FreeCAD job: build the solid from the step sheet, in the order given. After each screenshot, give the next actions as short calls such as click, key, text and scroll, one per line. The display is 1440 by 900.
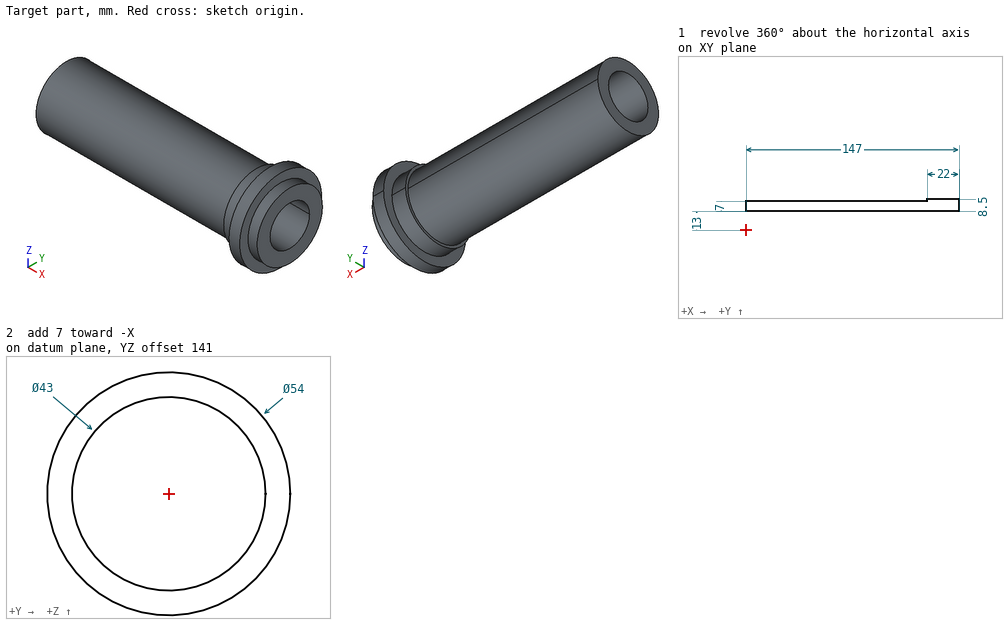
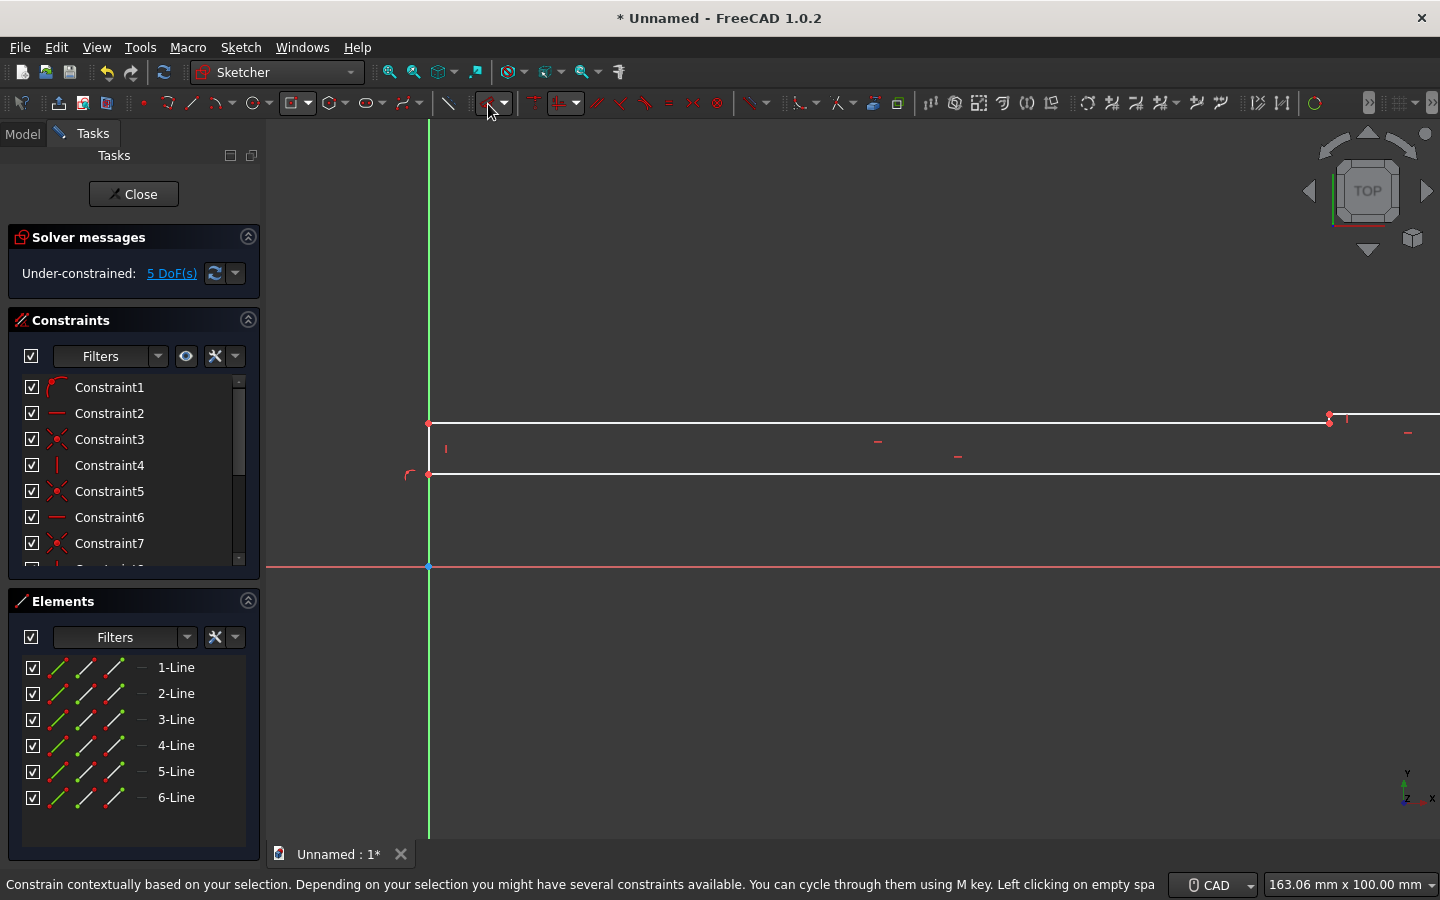
click(429, 438)
click(395, 449)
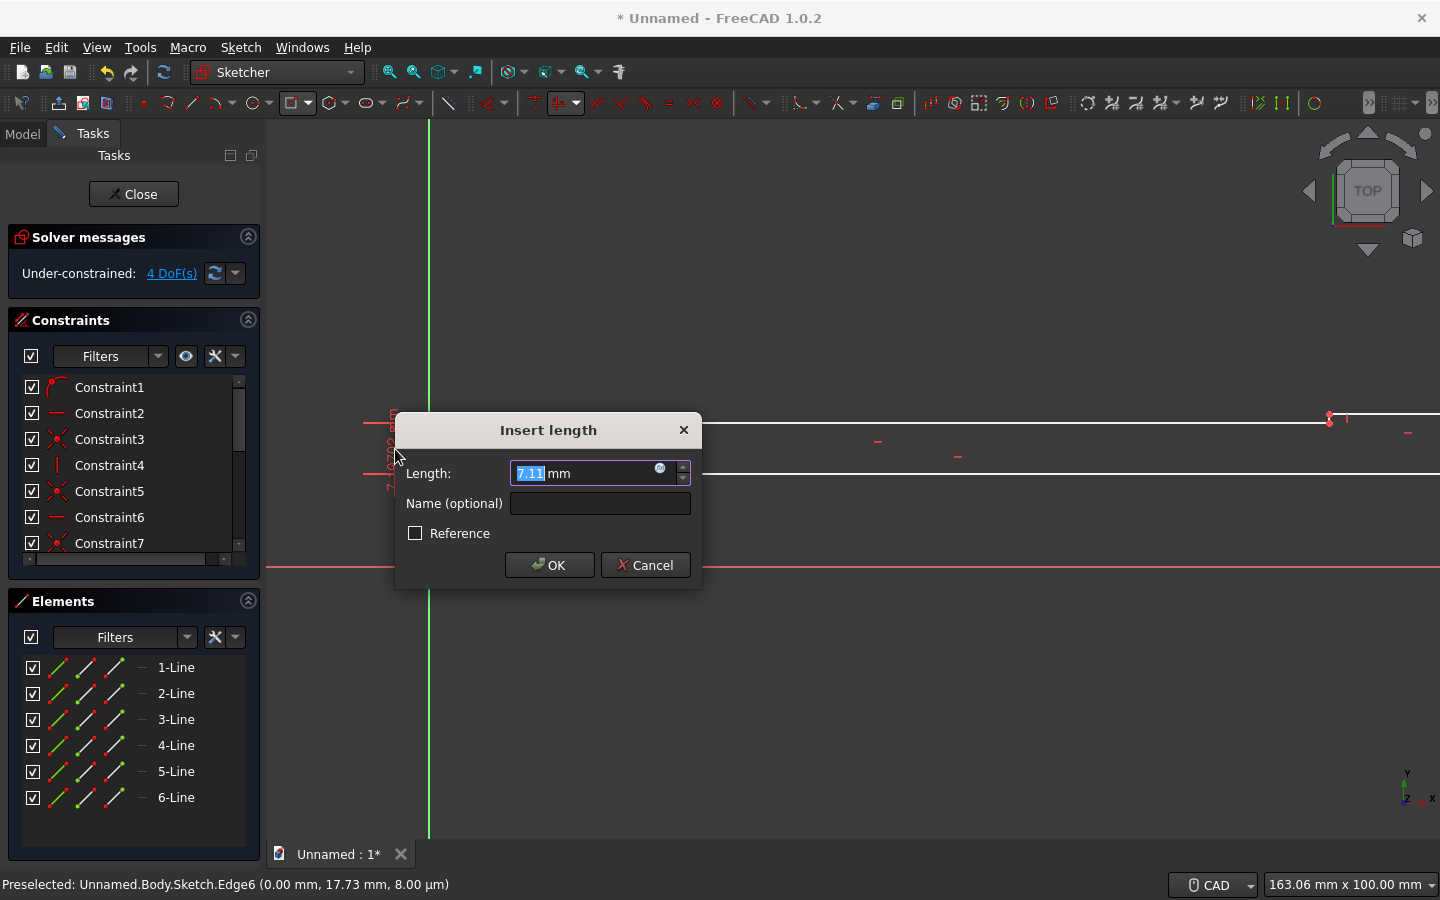
text(7)
key(Return)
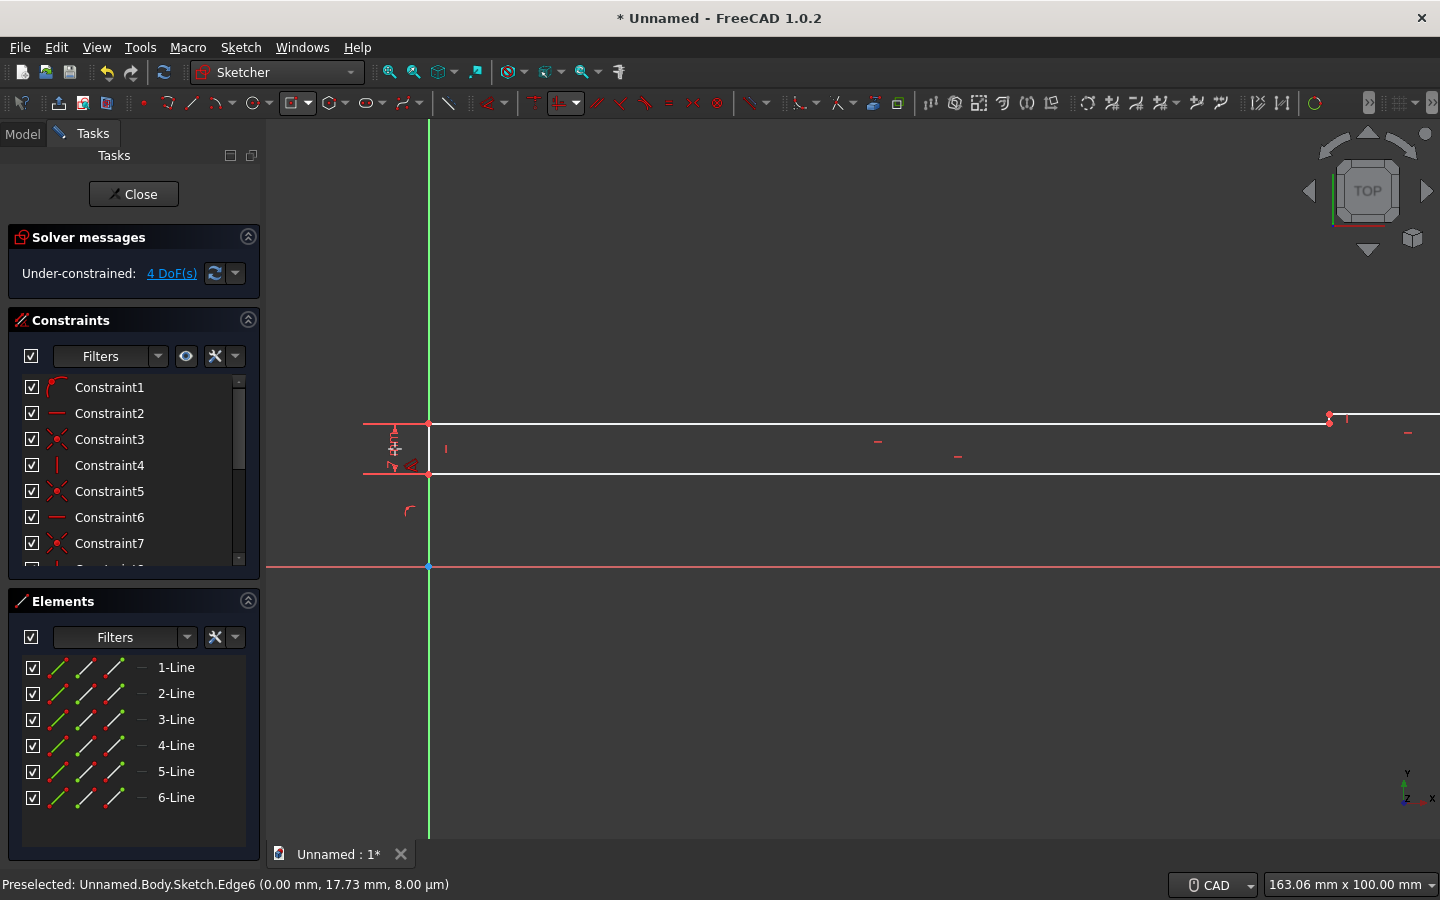
scroll(432, 458, down, 2)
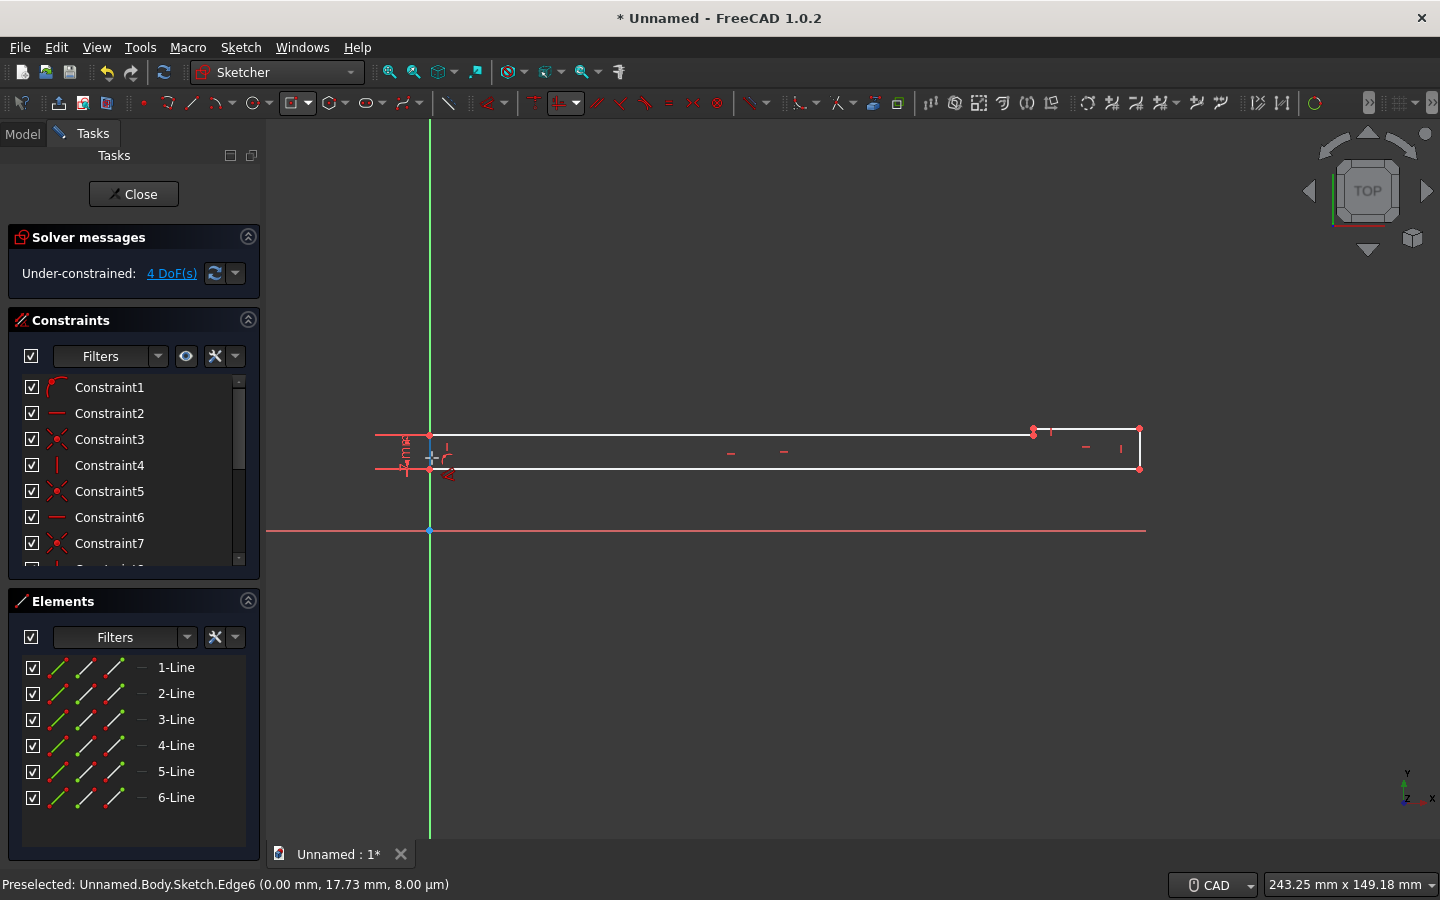
click(1108, 429)
click(1086, 395)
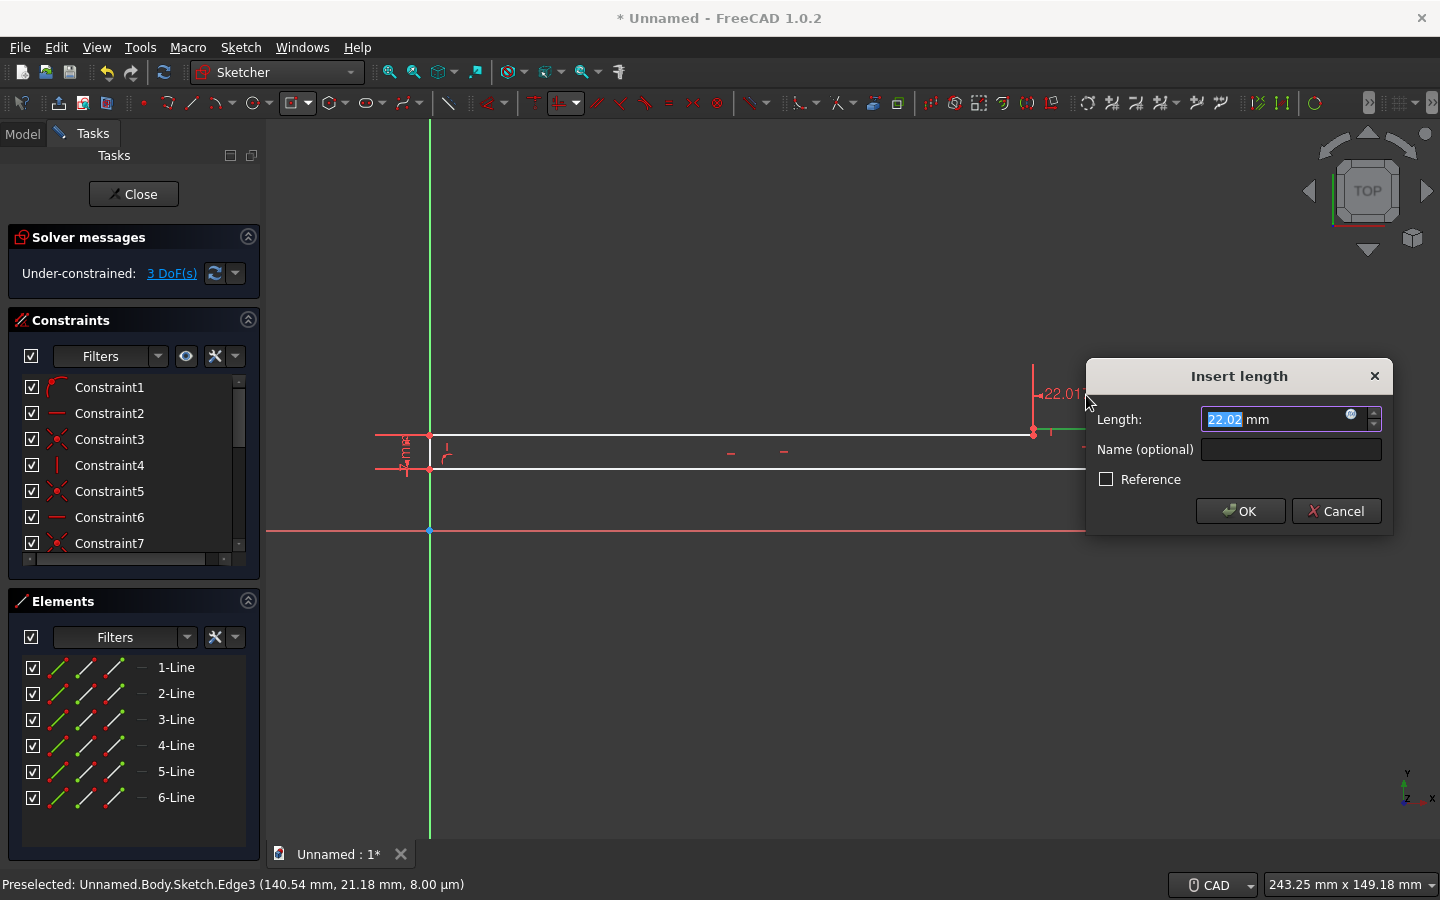
text(22)
key(Return)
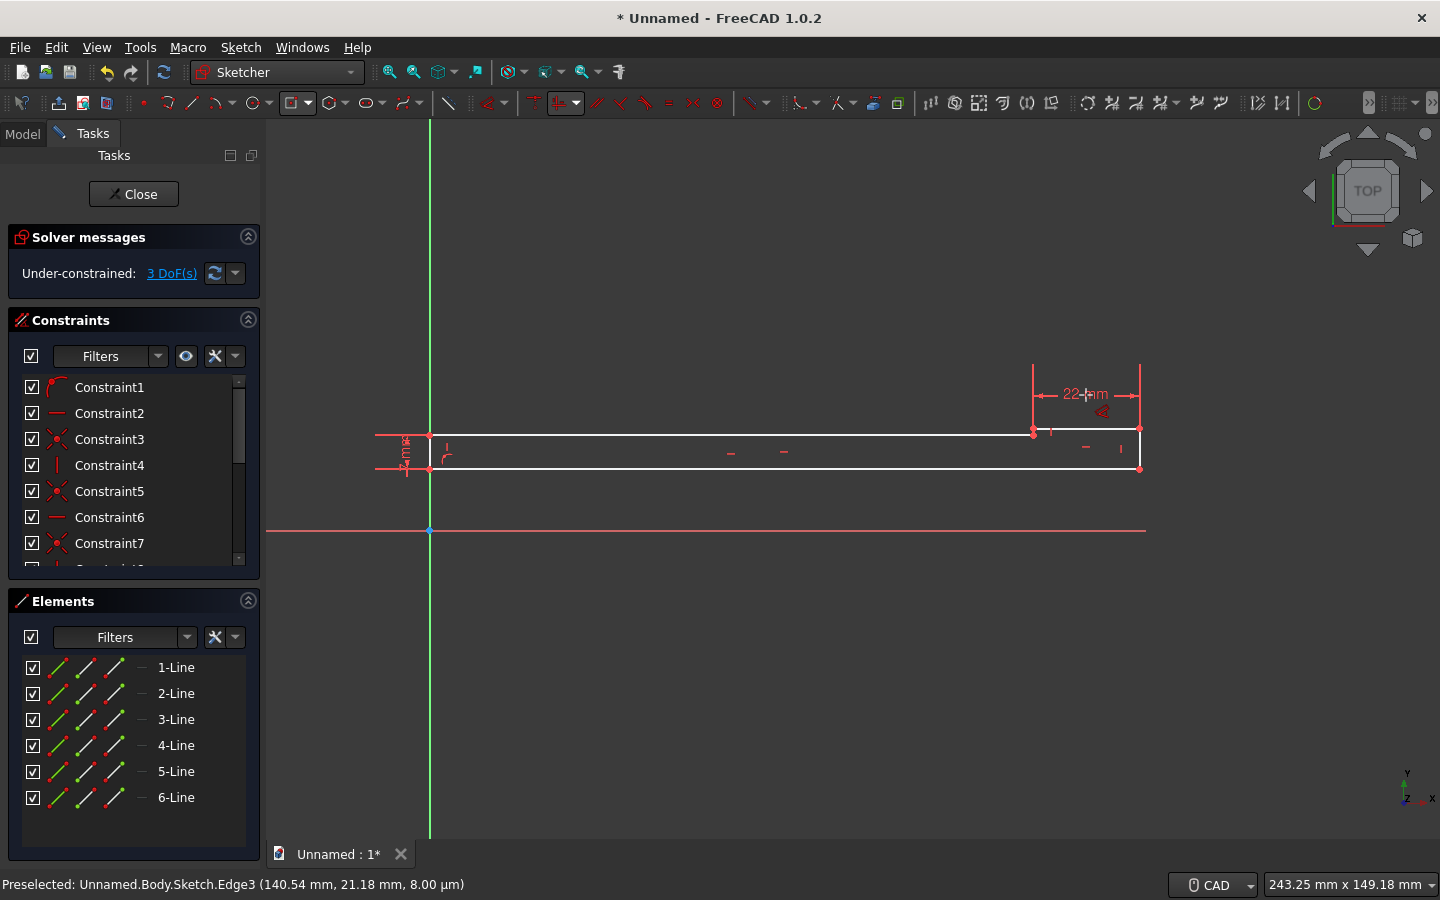
click(643, 469)
click(785, 503)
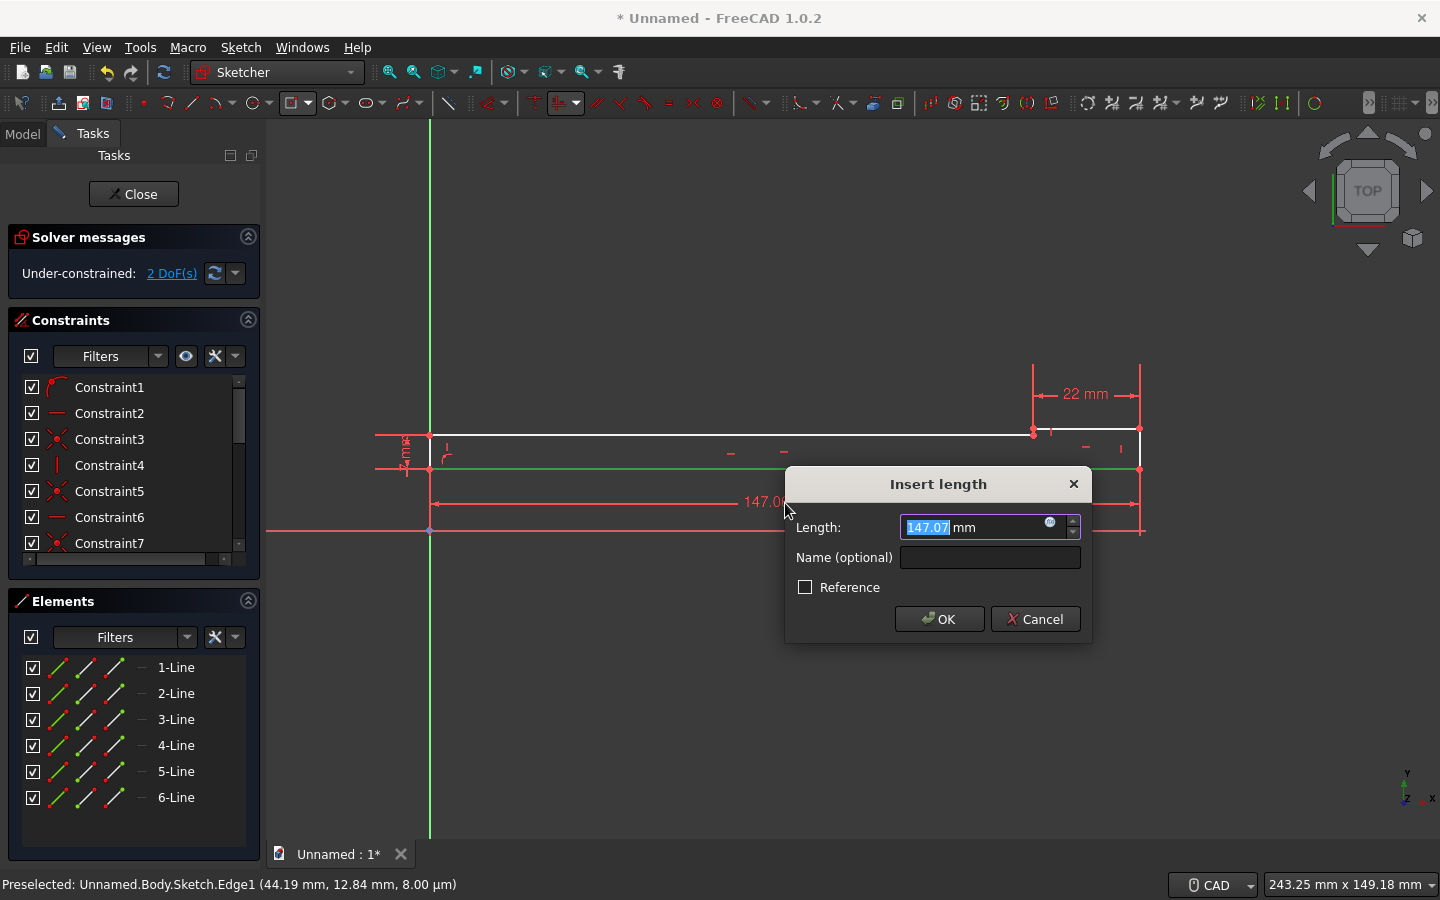
text(147)
key(Return)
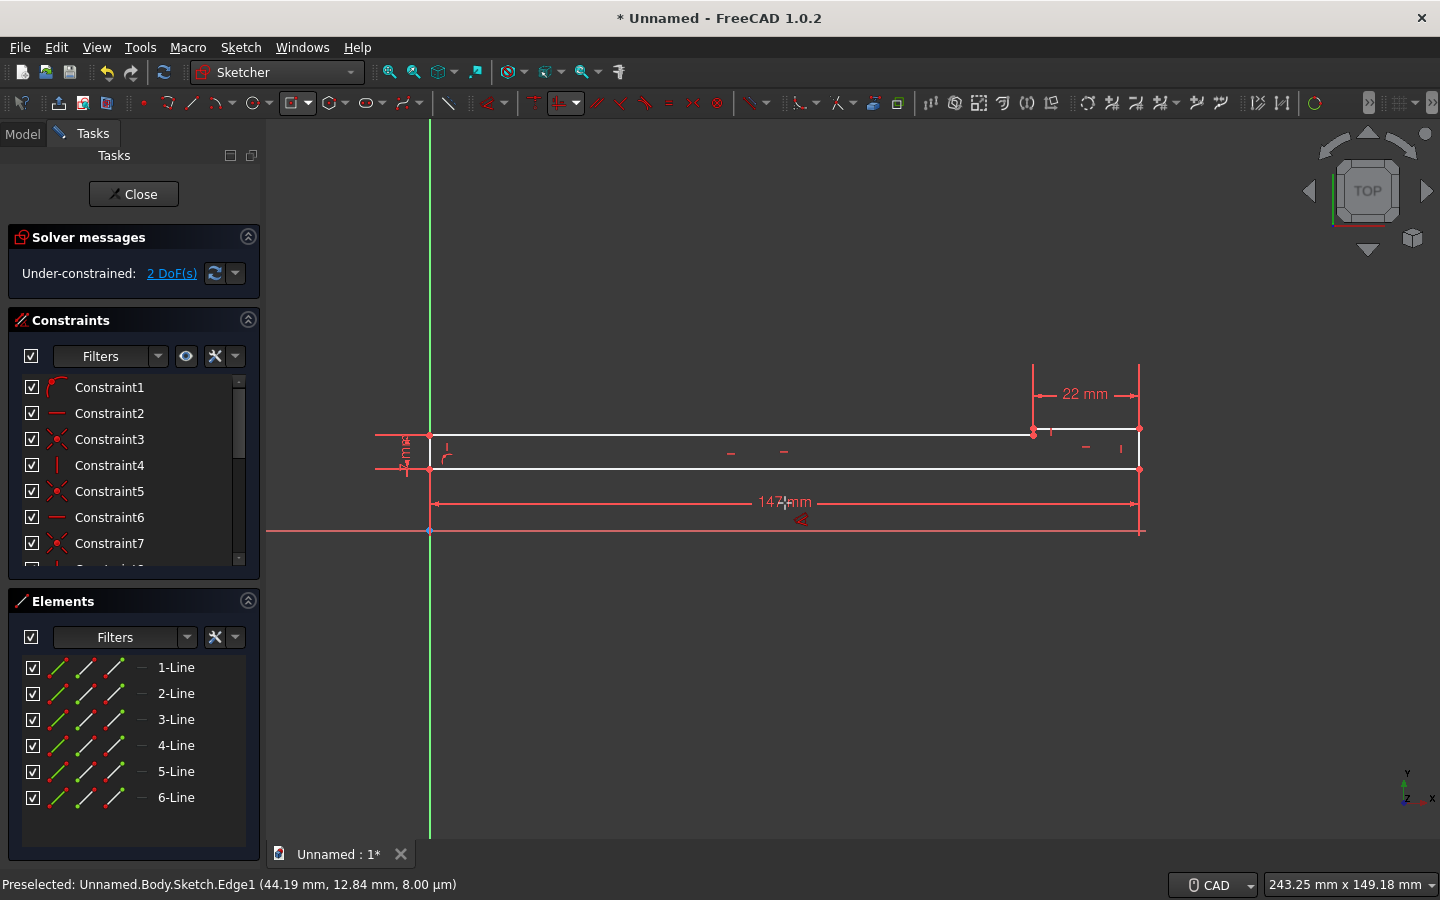
click(1139, 457)
click(1173, 449)